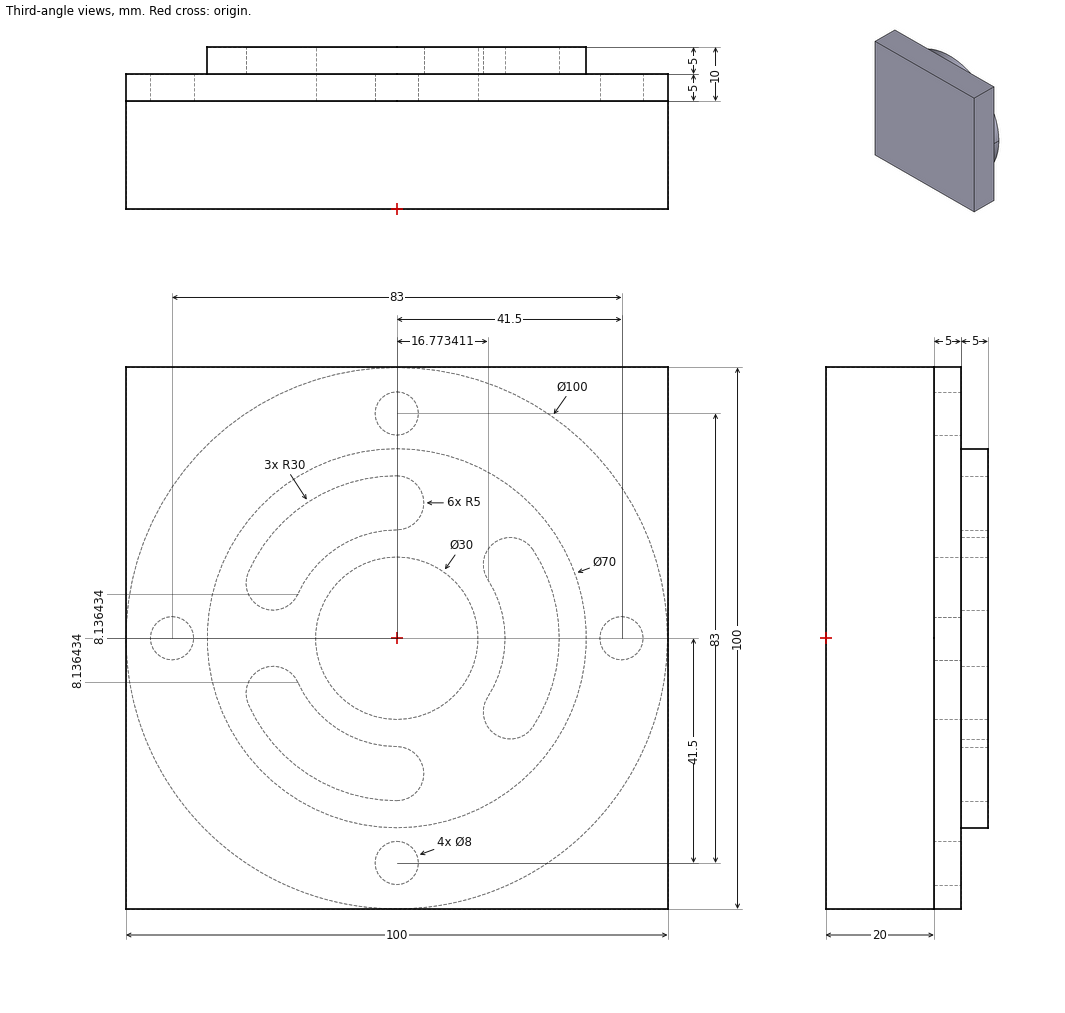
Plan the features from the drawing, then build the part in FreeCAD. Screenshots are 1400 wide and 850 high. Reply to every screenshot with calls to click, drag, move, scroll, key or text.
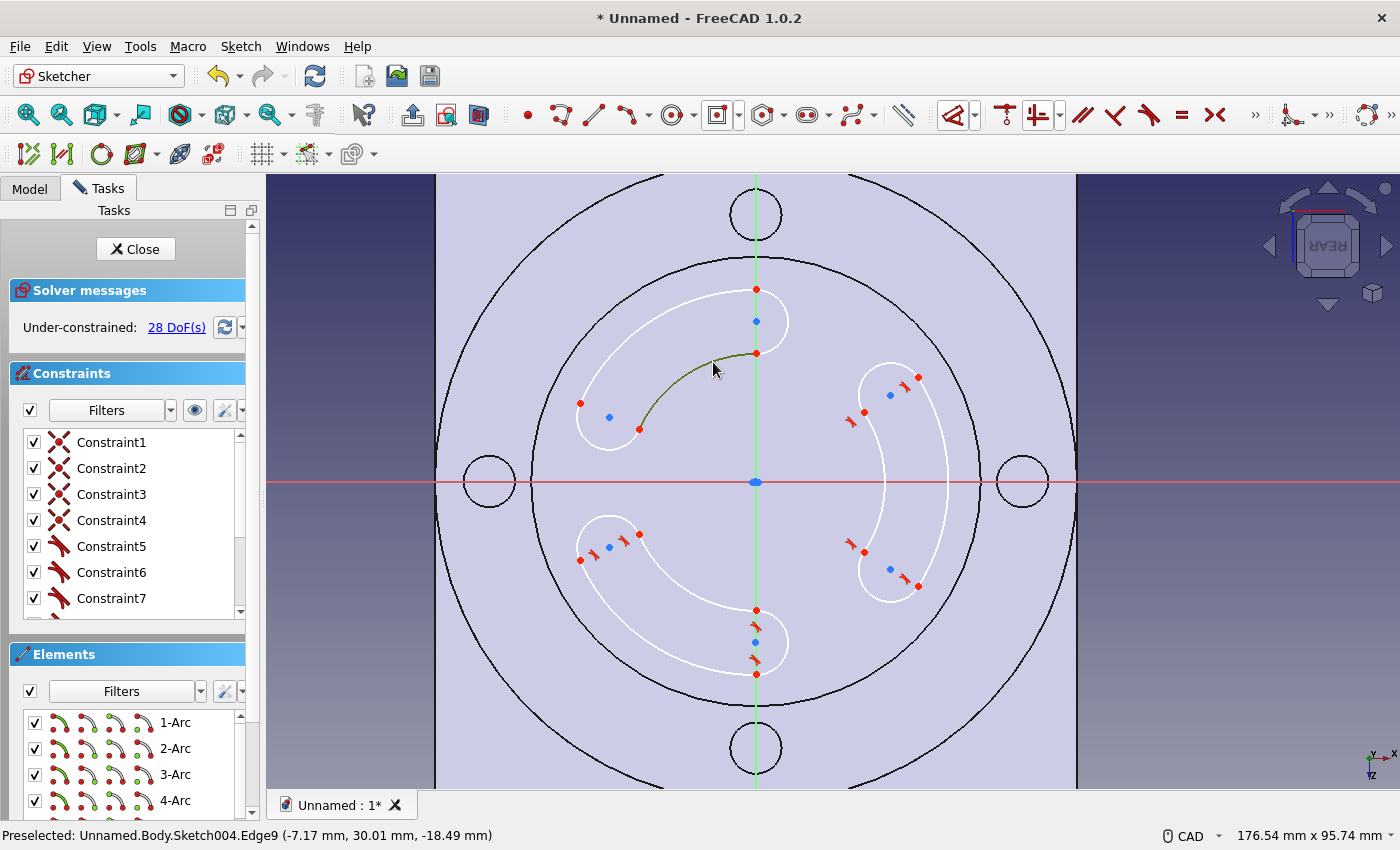
click(782, 341)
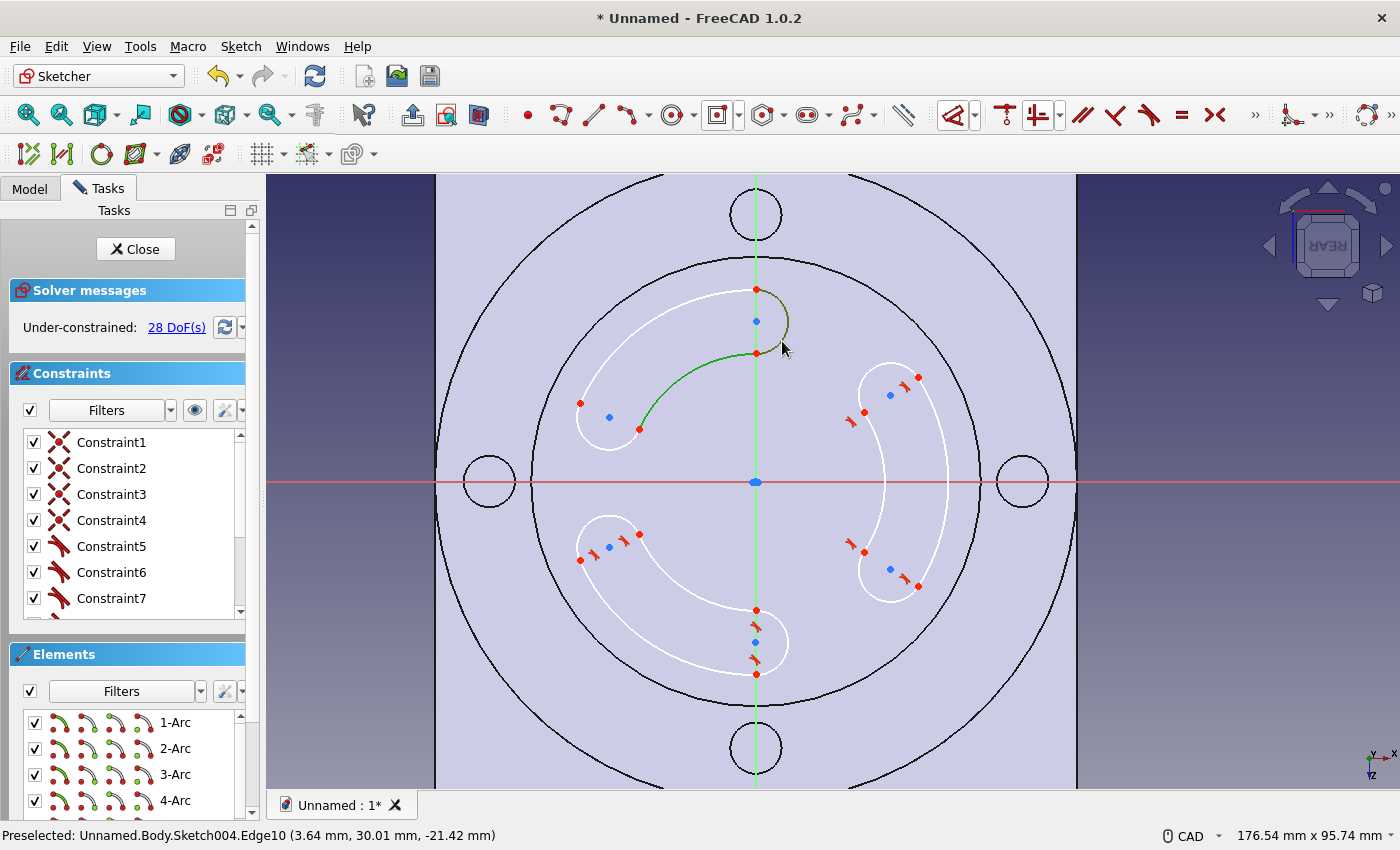
click(1149, 116)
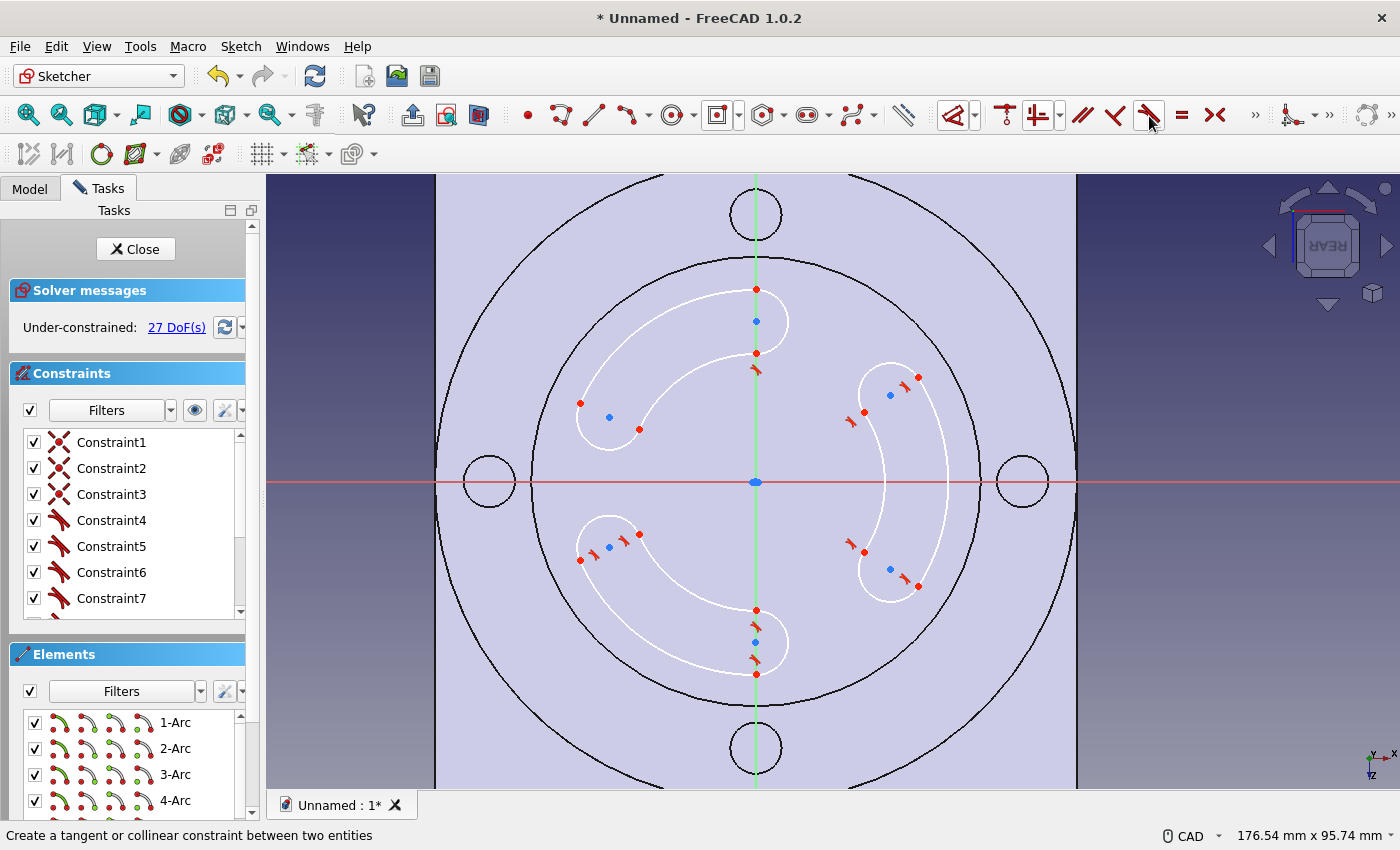
click(713, 362)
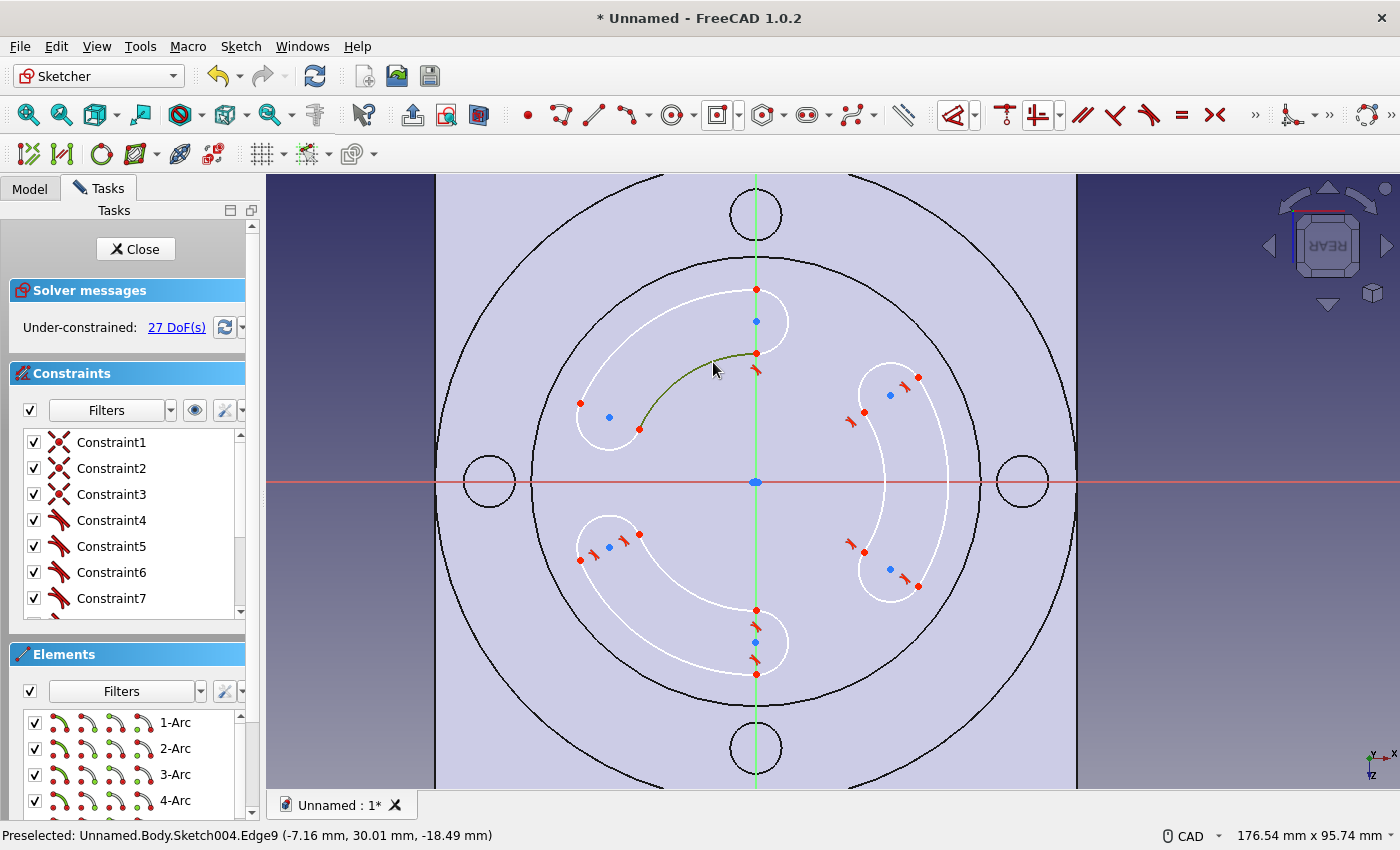
click(581, 434)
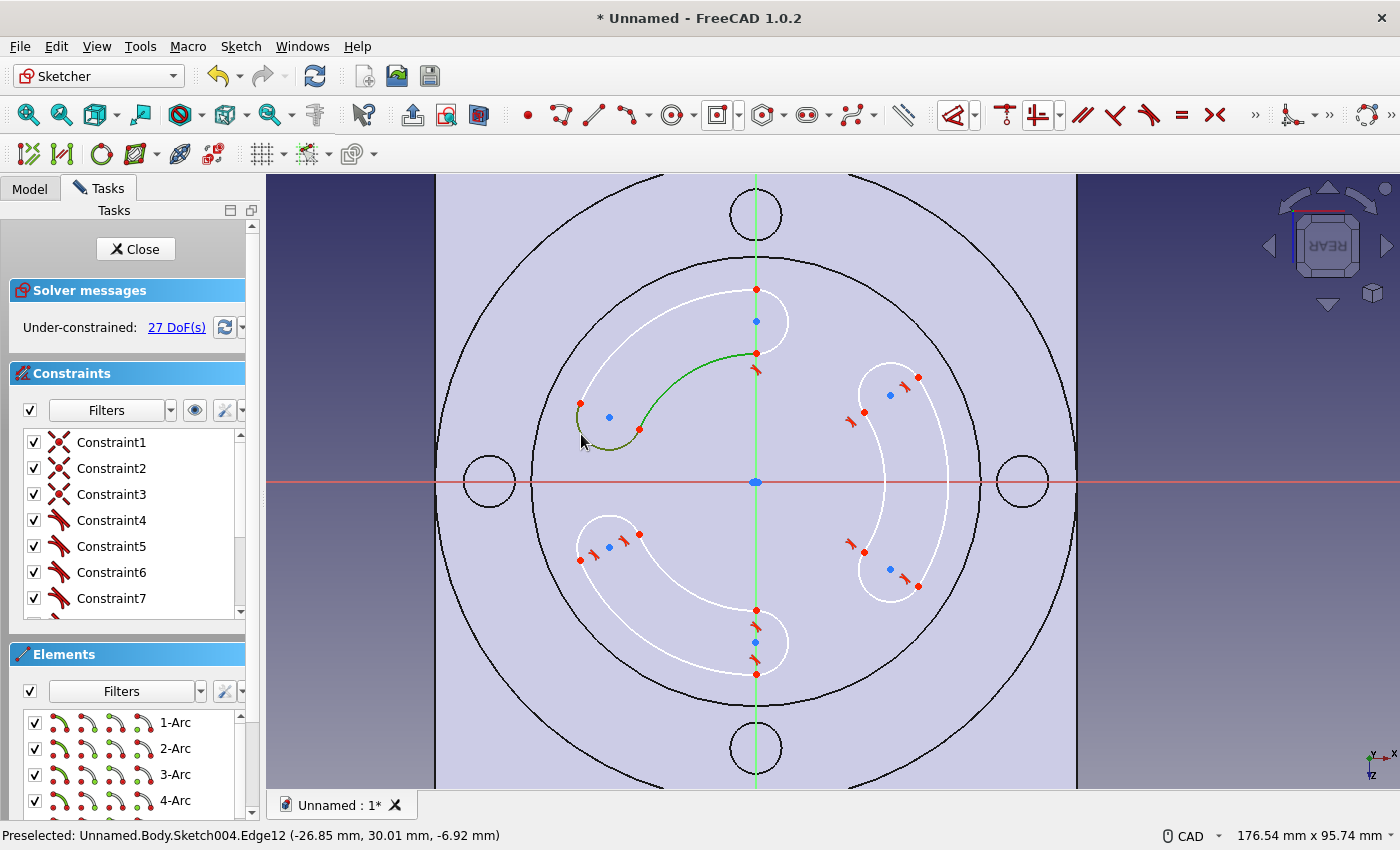
click(1149, 116)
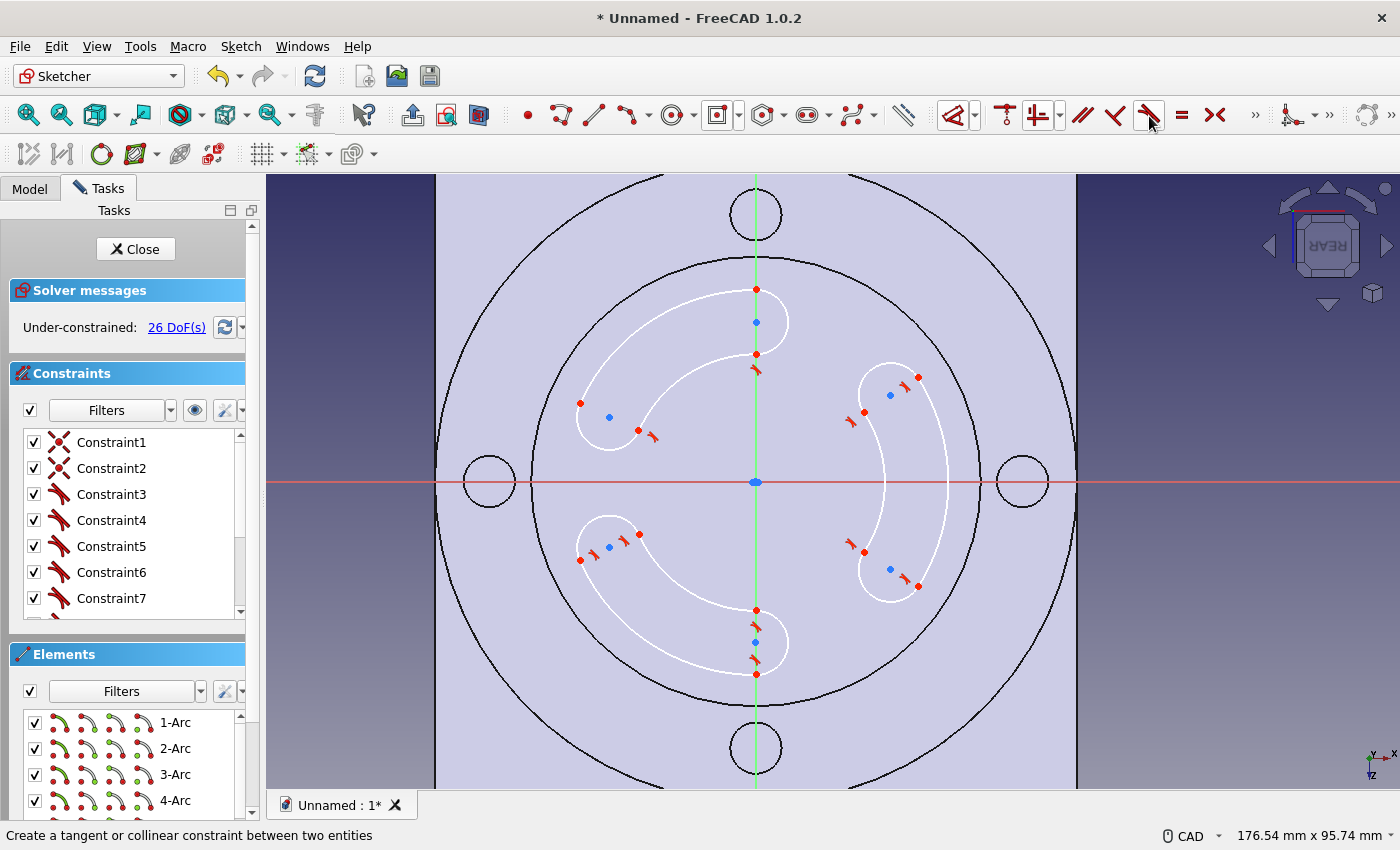
click(782, 341)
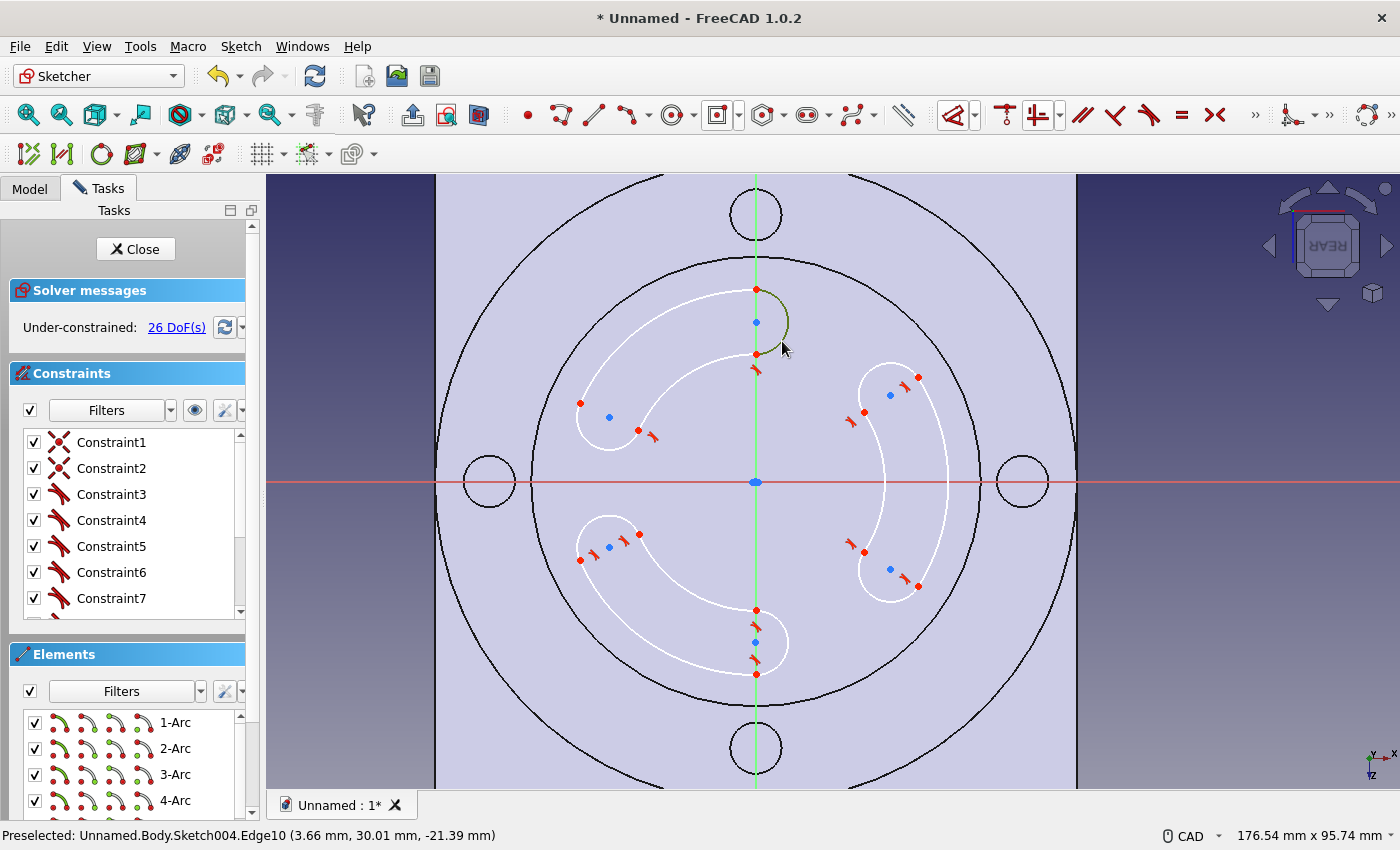
click(691, 301)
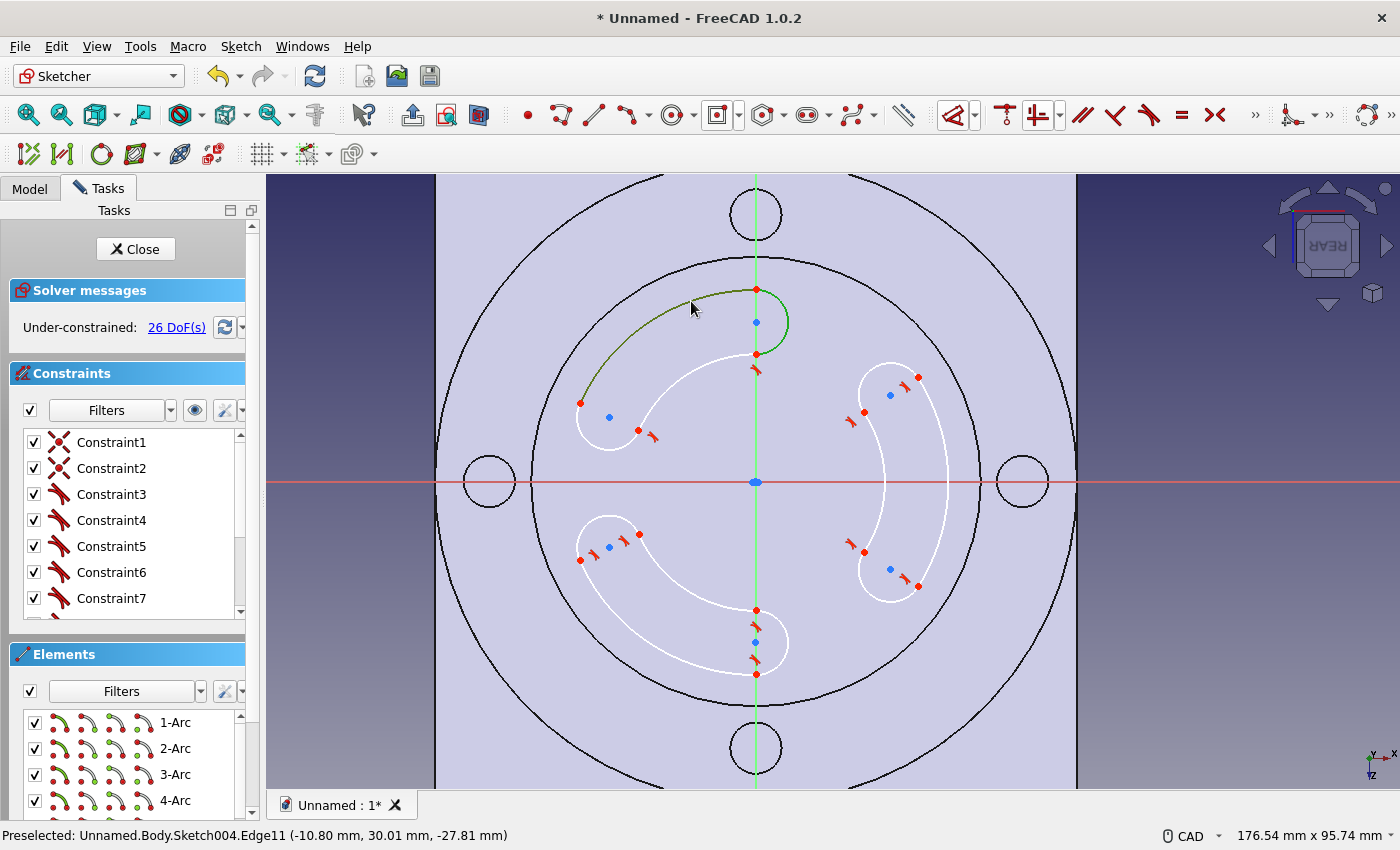
click(1149, 116)